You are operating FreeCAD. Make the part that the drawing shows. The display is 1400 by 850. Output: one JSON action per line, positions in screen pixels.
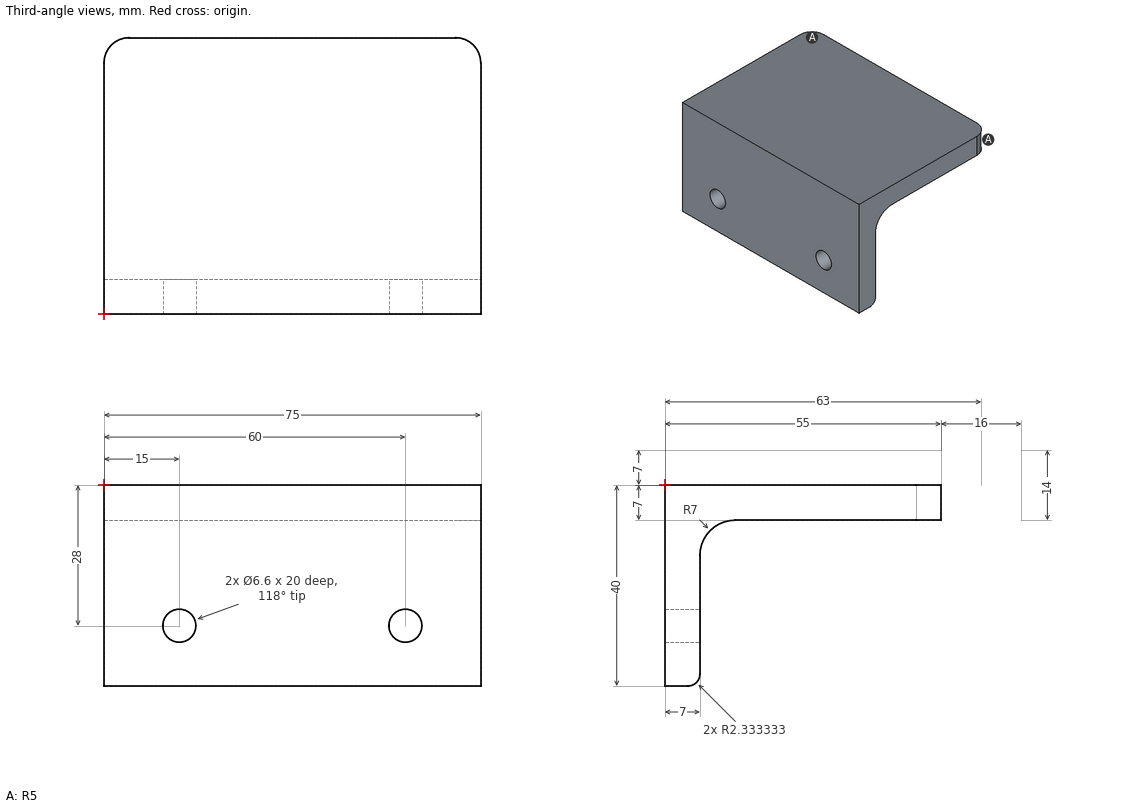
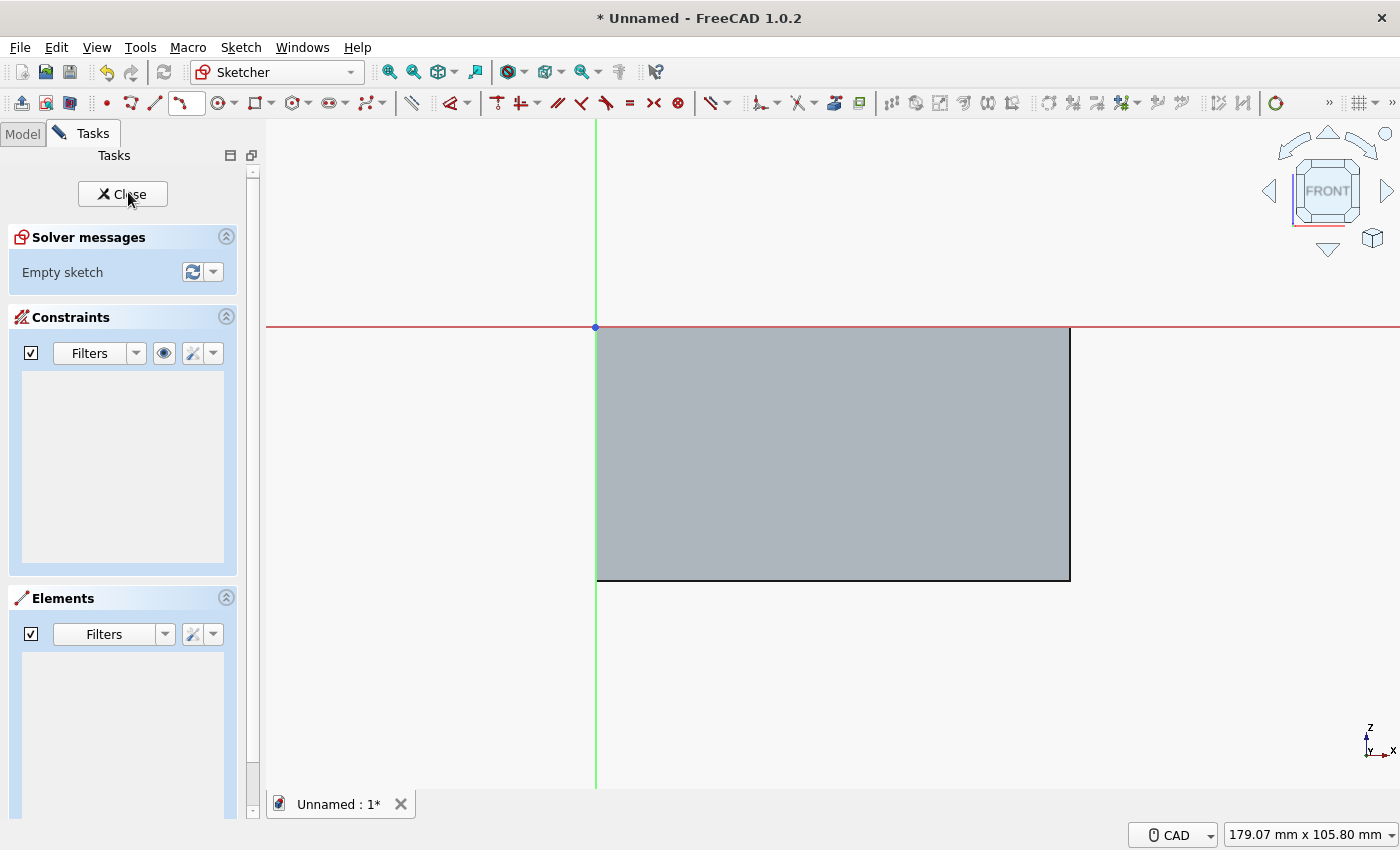
{"action": "scroll", "coordinate": [834, 393], "scroll_direction": "up", "scroll_amount": 3}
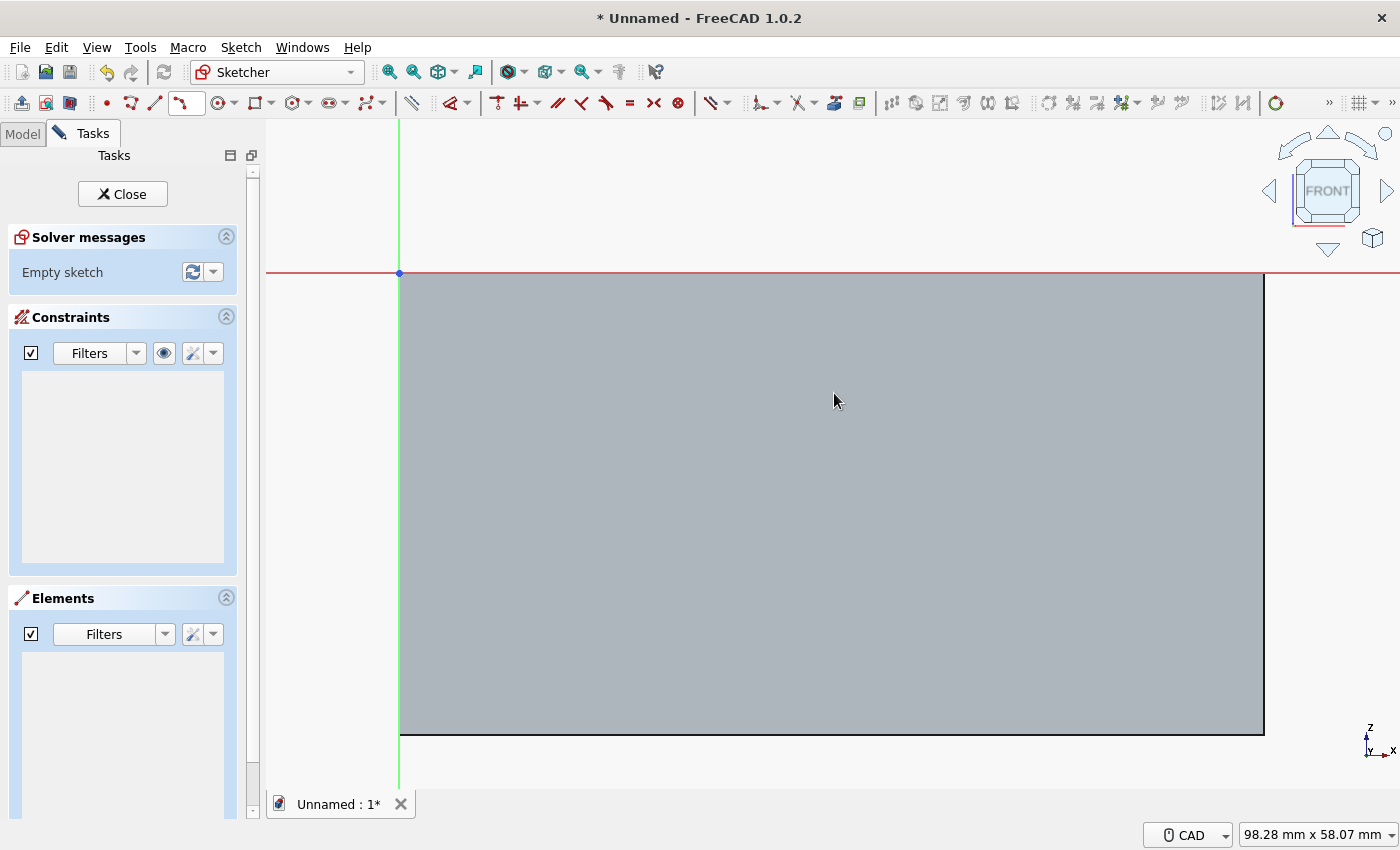
{"action": "left_click", "coordinate": [218, 104]}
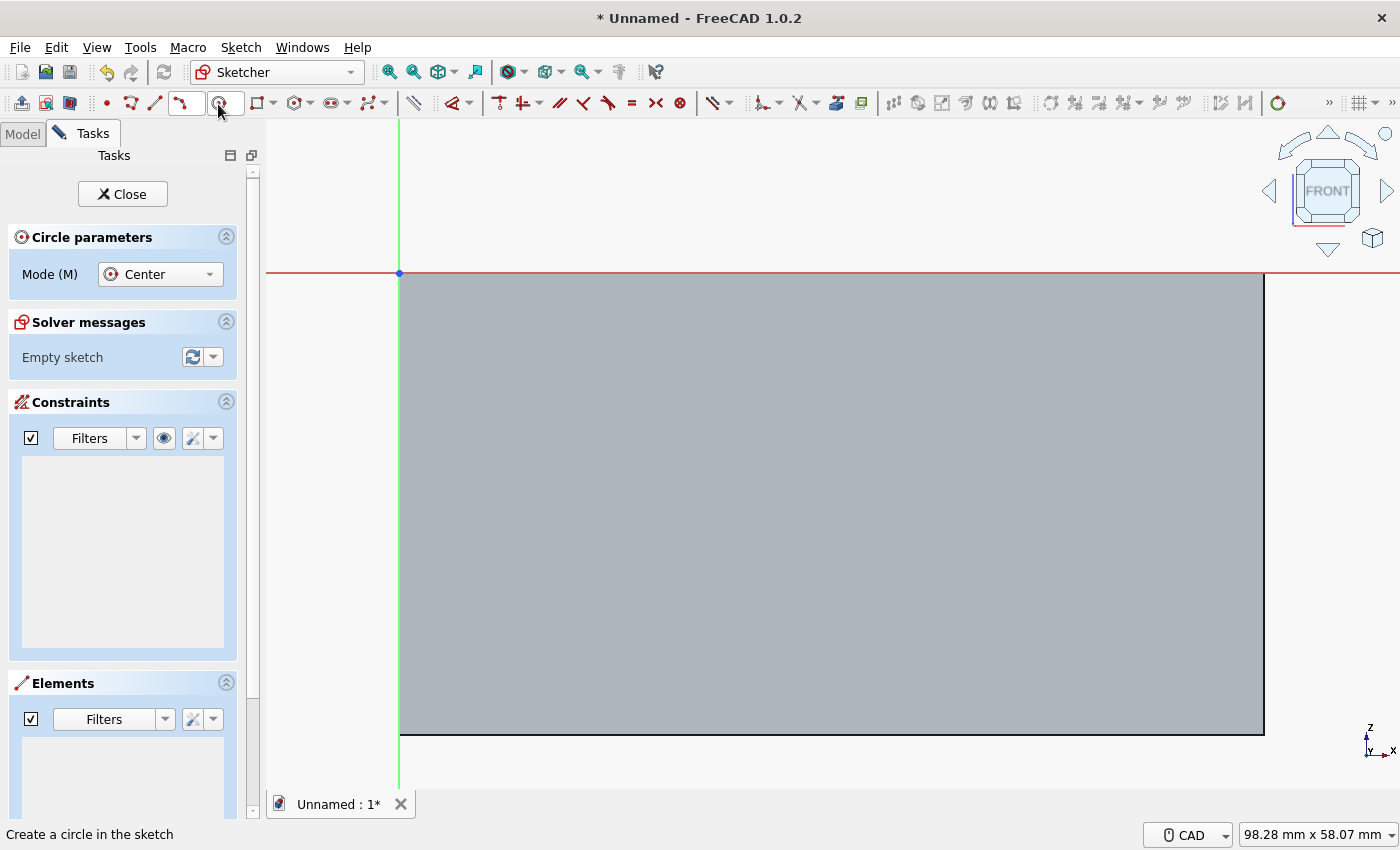
{"action": "left_click", "coordinate": [572, 596]}
{"action": "mouse_move", "coordinate": [599, 569]}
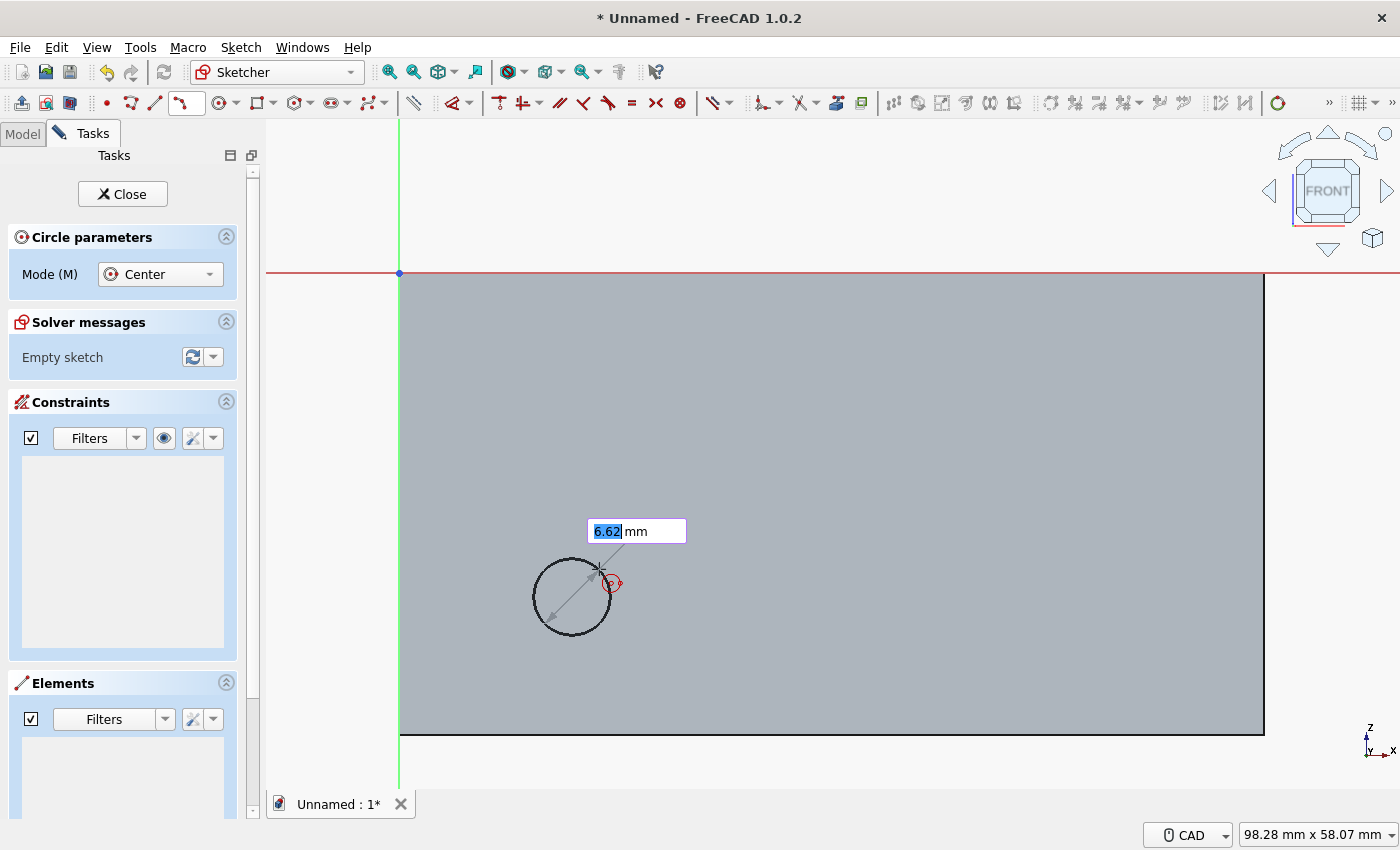
{"action": "type", "text": "6.6"}
{"action": "key", "text": "Return"}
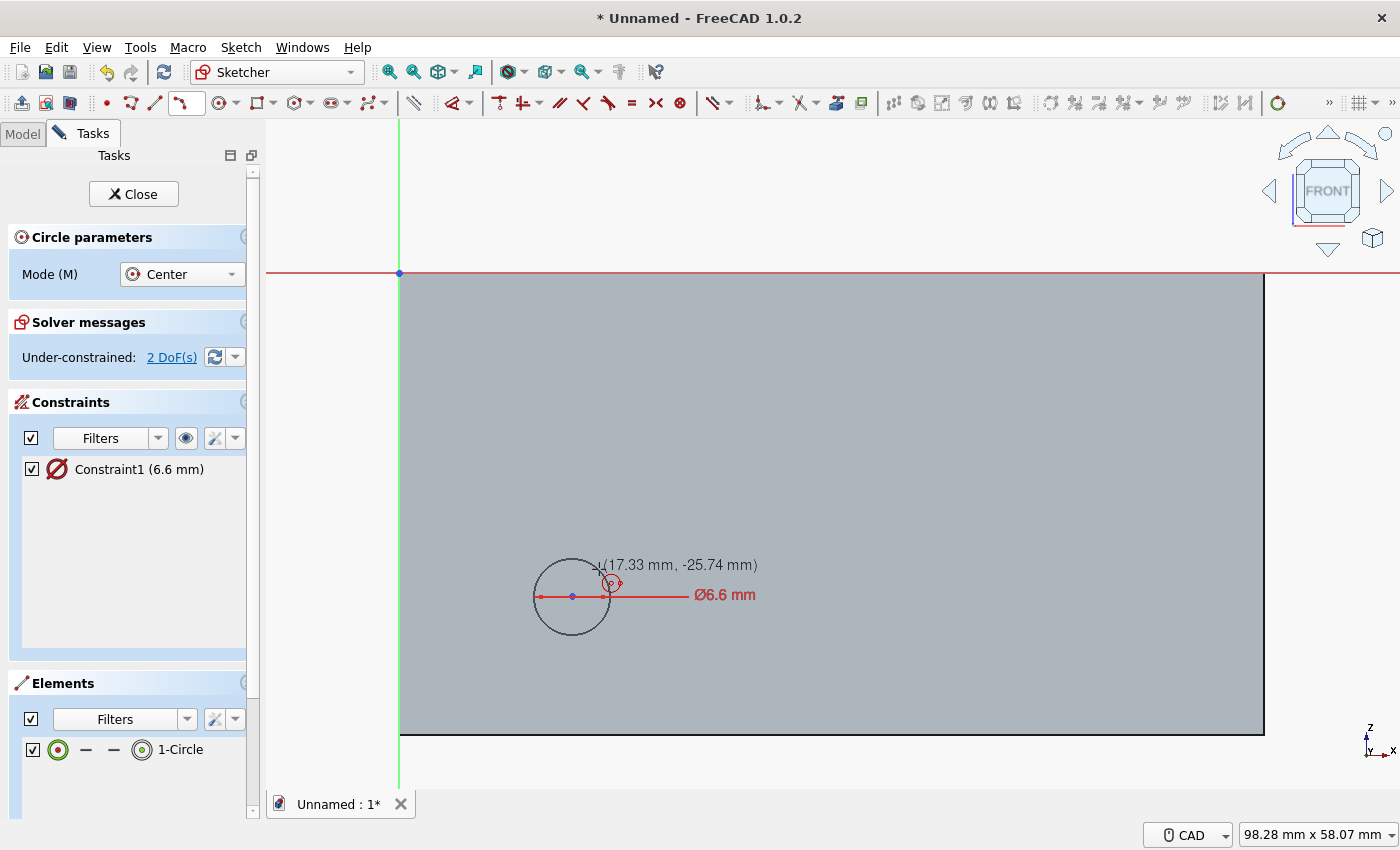
{"action": "left_click", "coordinate": [1091, 596]}
{"action": "mouse_move", "coordinate": [1118, 569]}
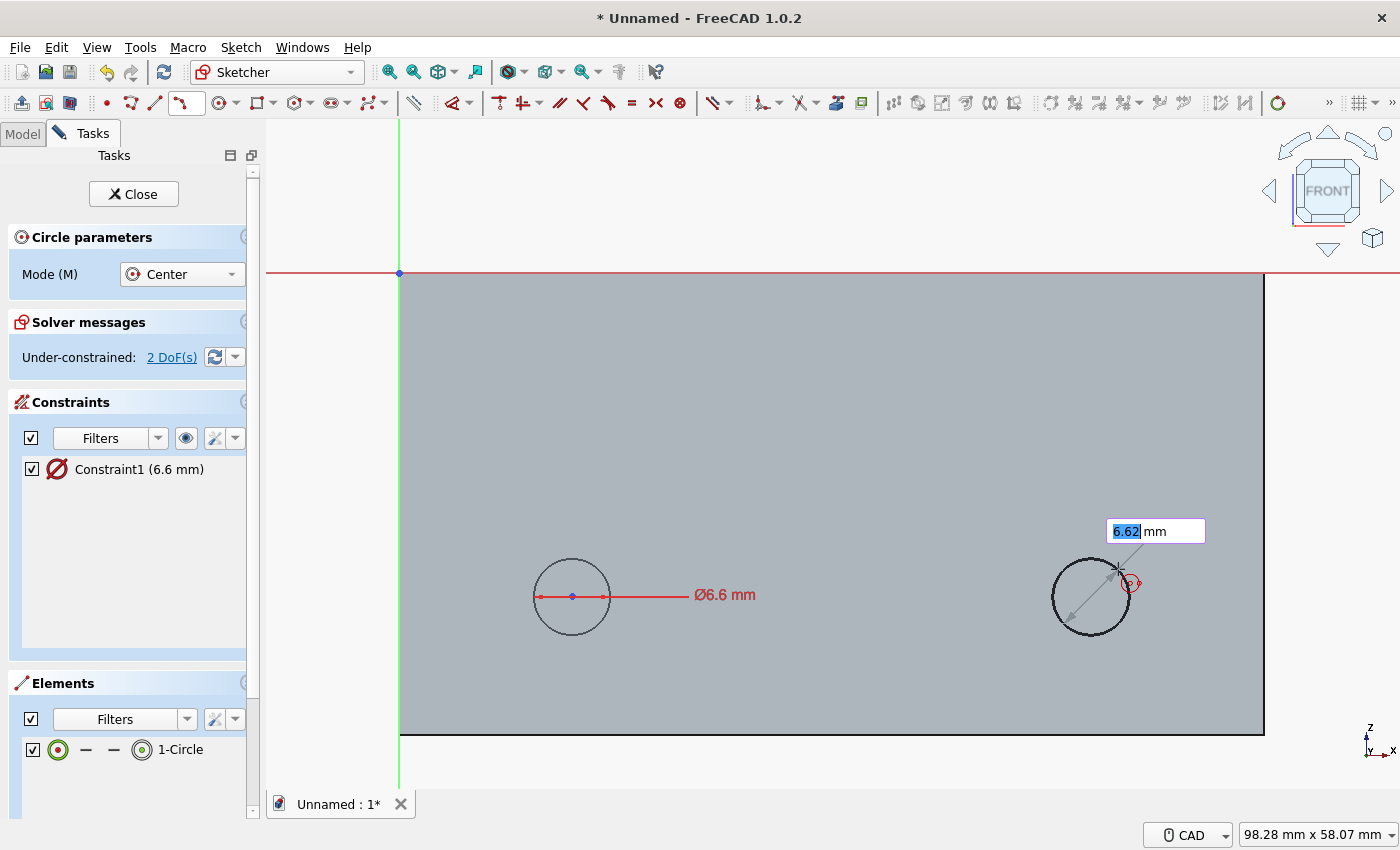
{"action": "type", "text": "6.6"}
{"action": "key", "text": "Return"}
{"action": "key", "text": "Escape"}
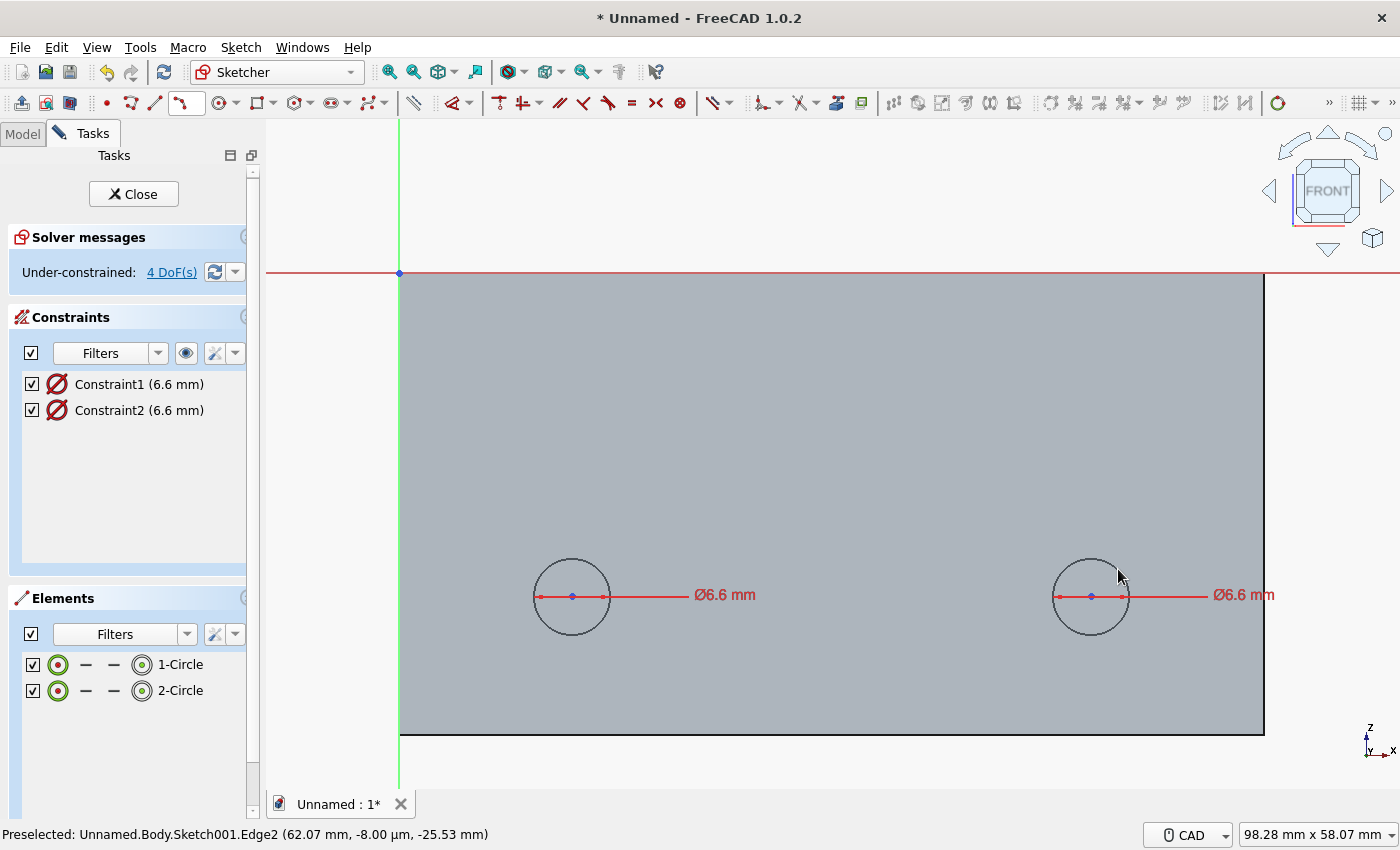
{"action": "left_click", "coordinate": [572, 597]}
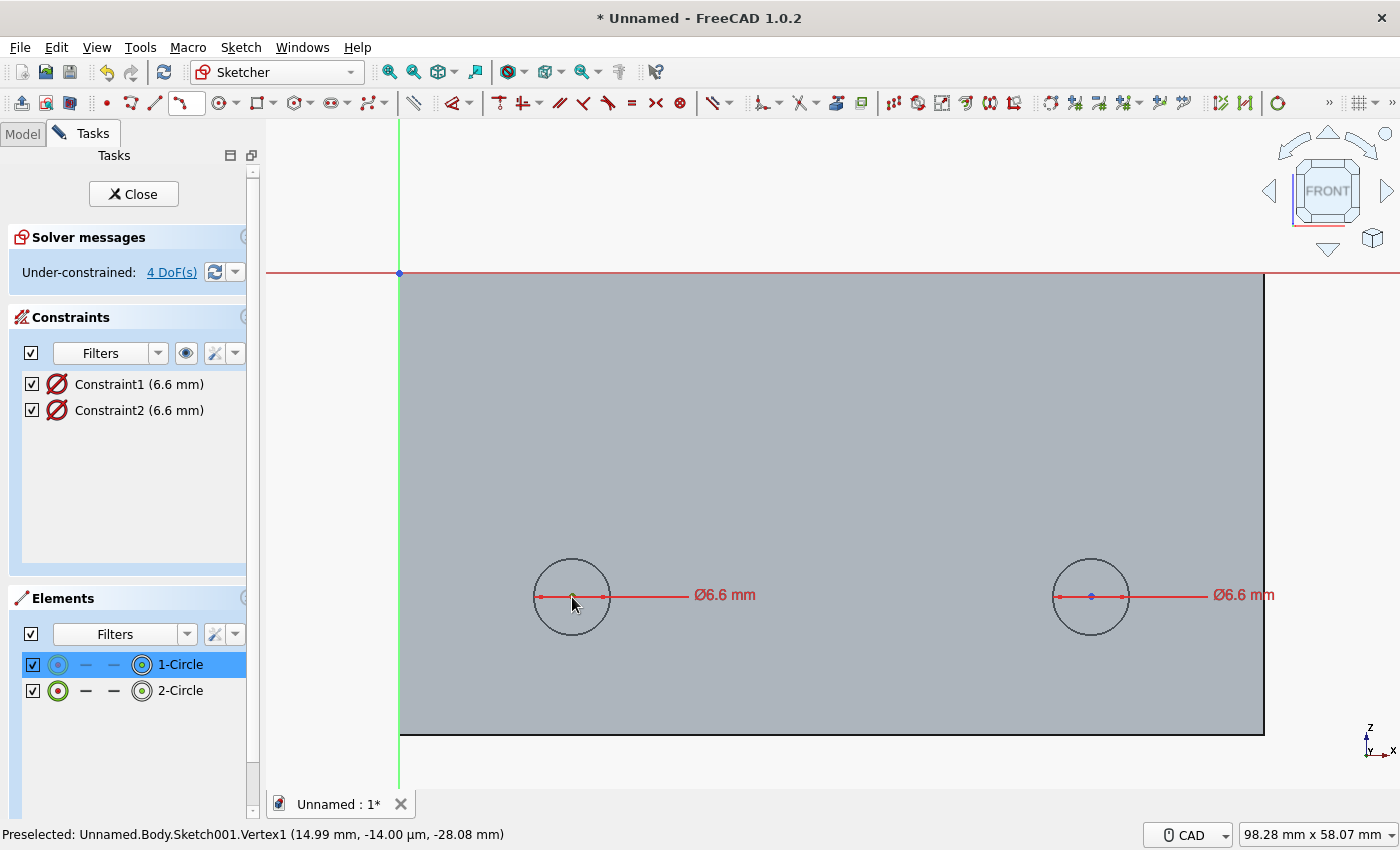
{"action": "left_click", "coordinate": [1091, 597]}